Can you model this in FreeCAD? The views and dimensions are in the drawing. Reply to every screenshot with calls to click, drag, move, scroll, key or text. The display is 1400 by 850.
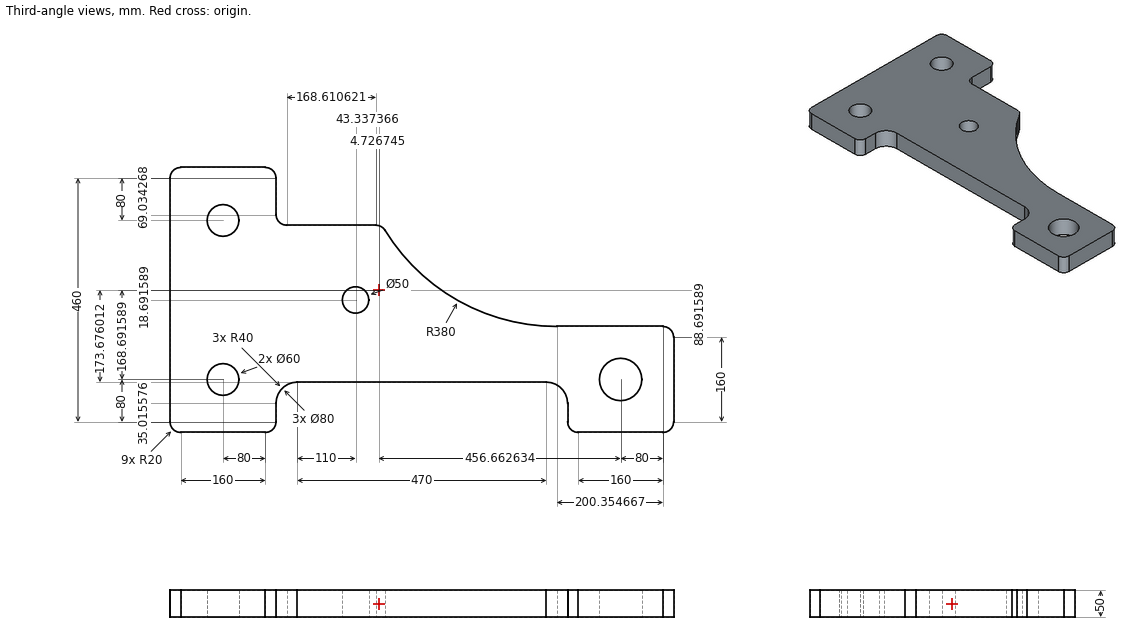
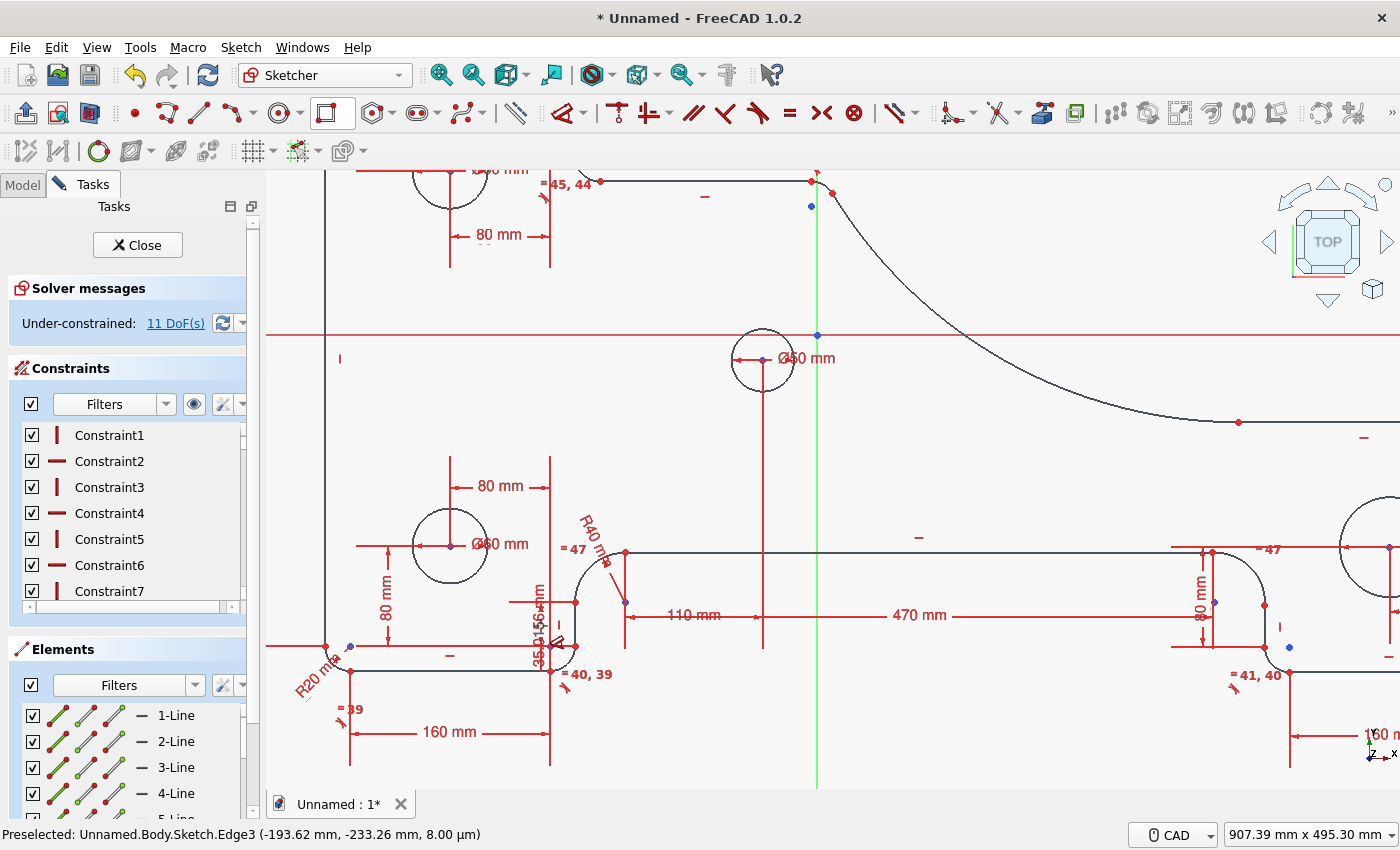
scroll(576, 626, down, 3)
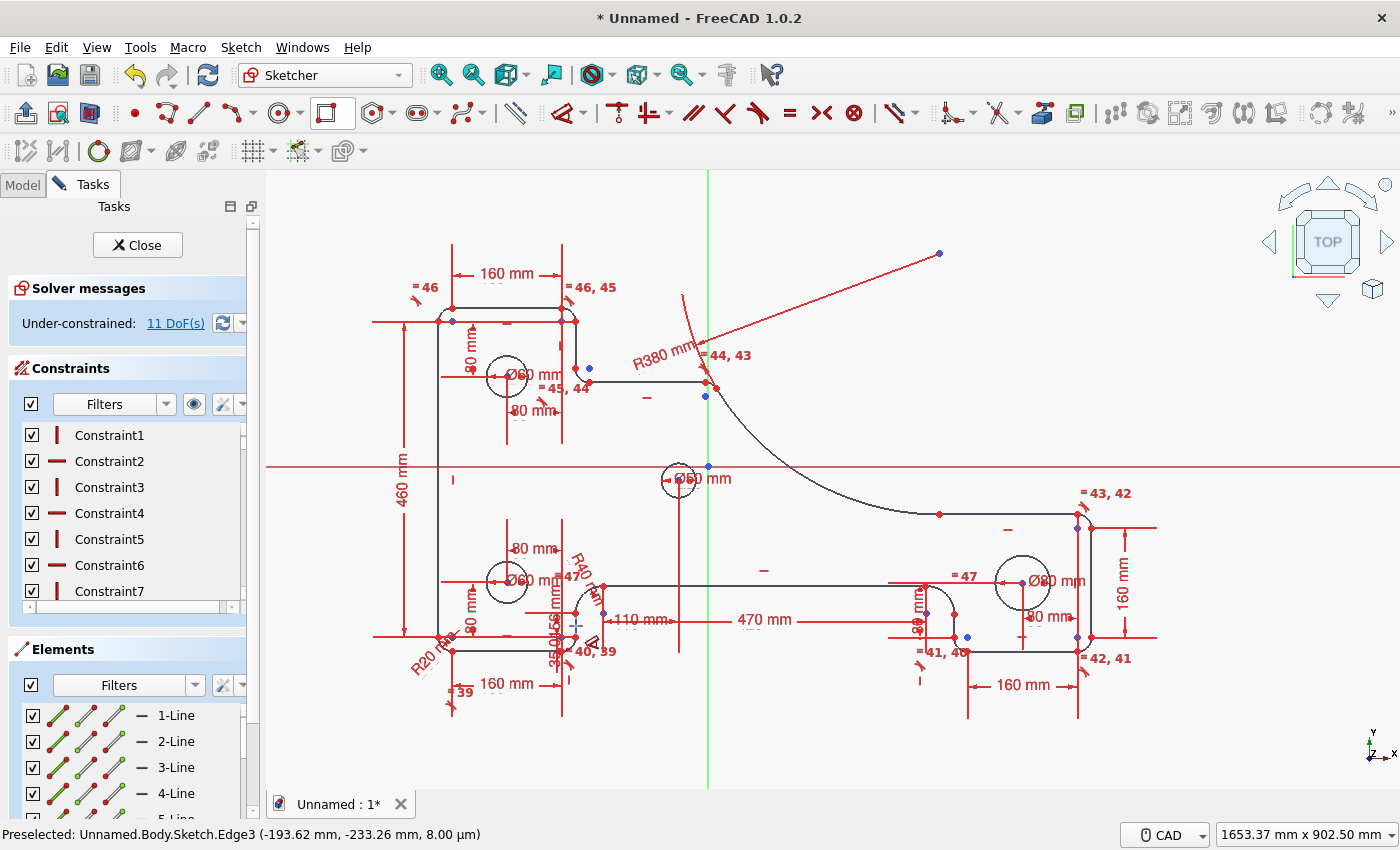
scroll(954, 622, up, 4)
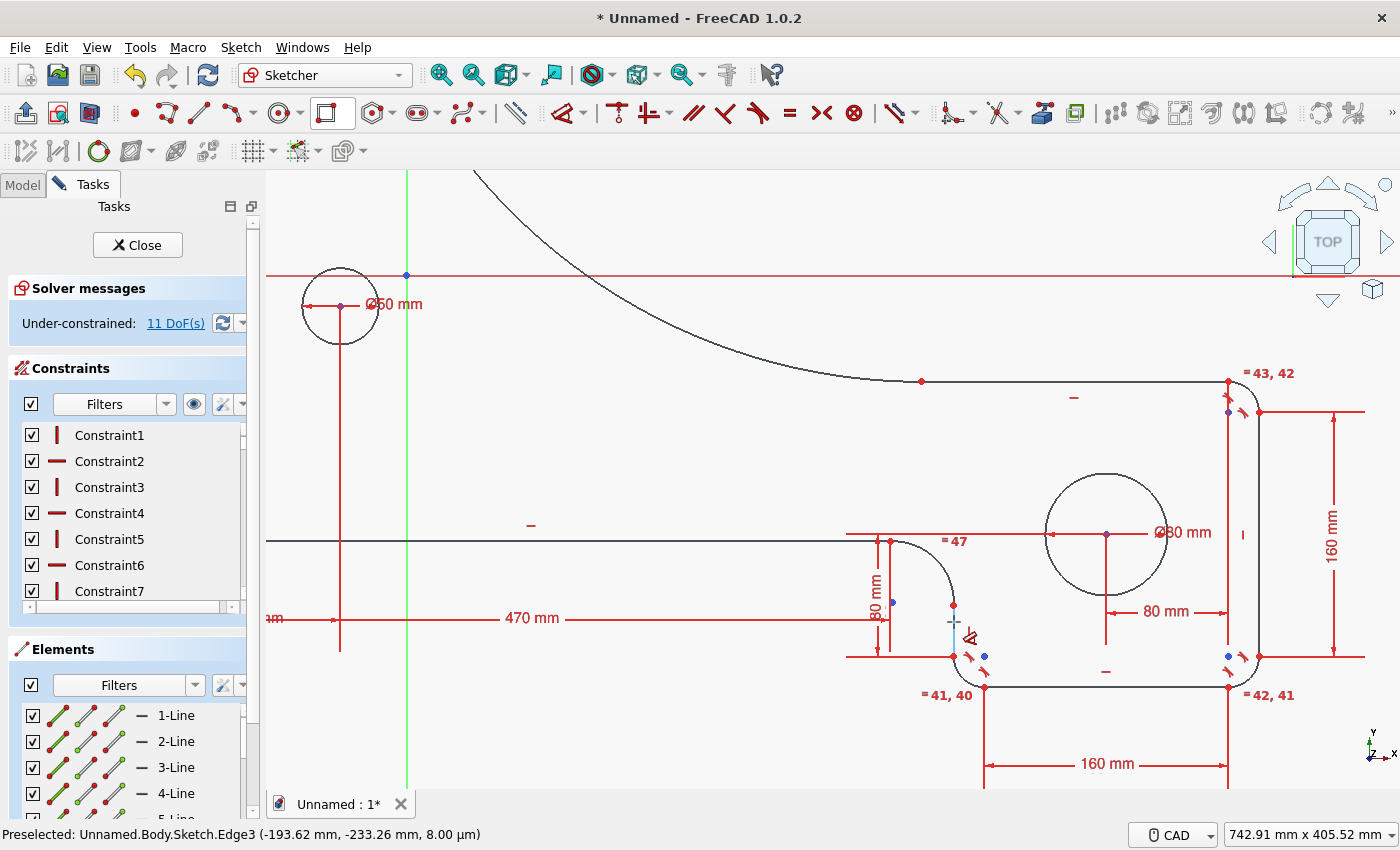
click(954, 621)
click(988, 631)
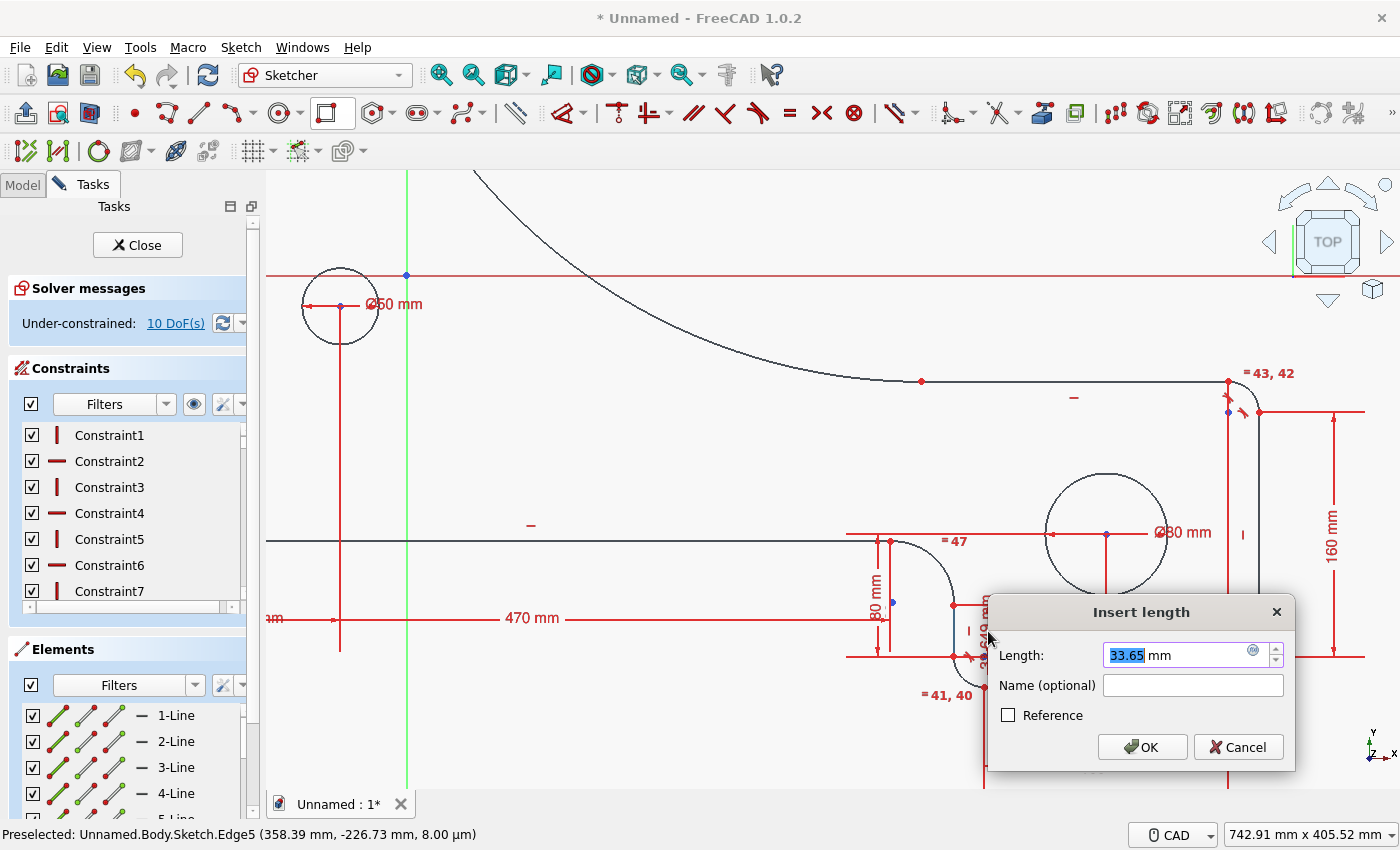
text(35.015576)
key(Return)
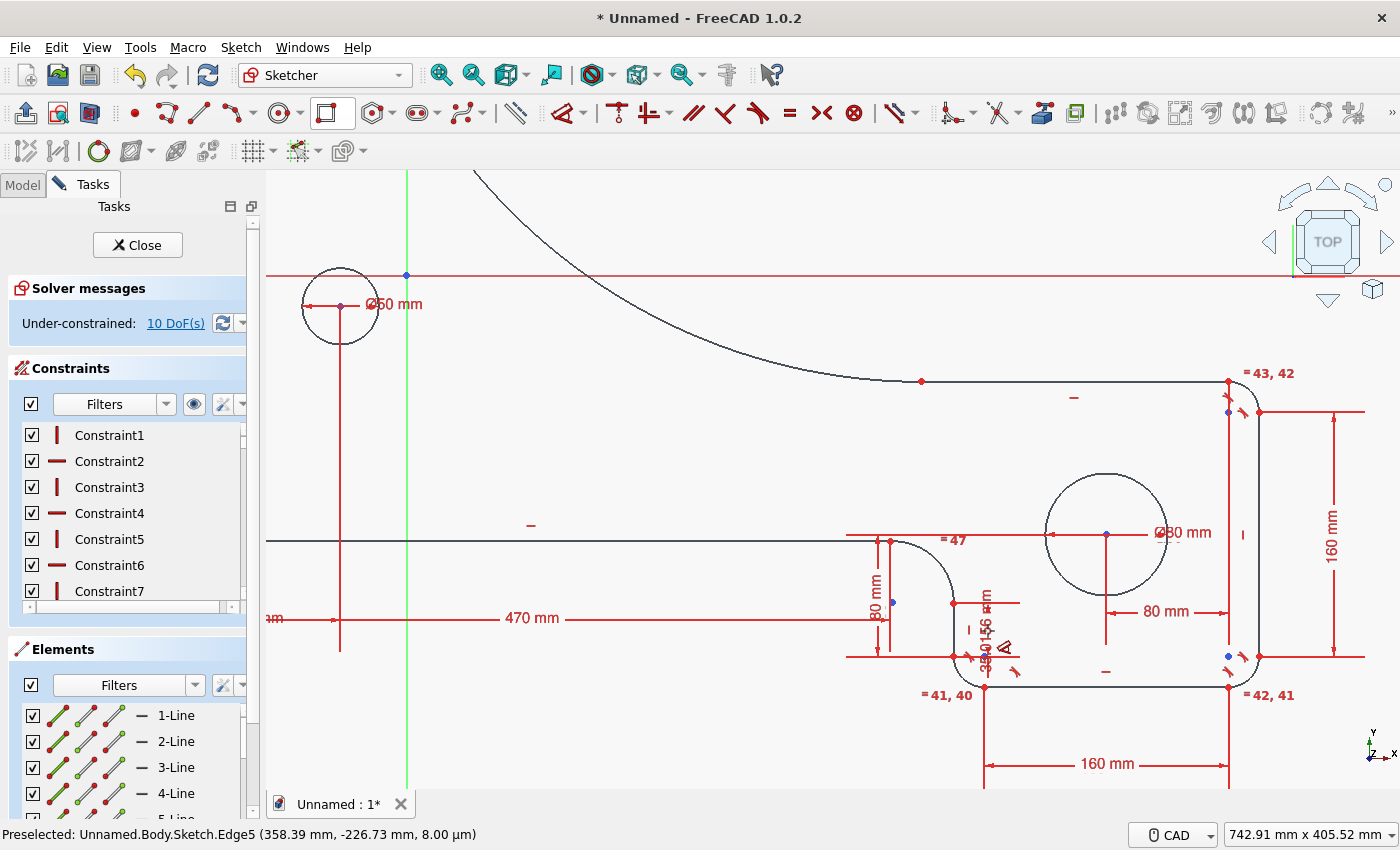
scroll(955, 622, down, 4)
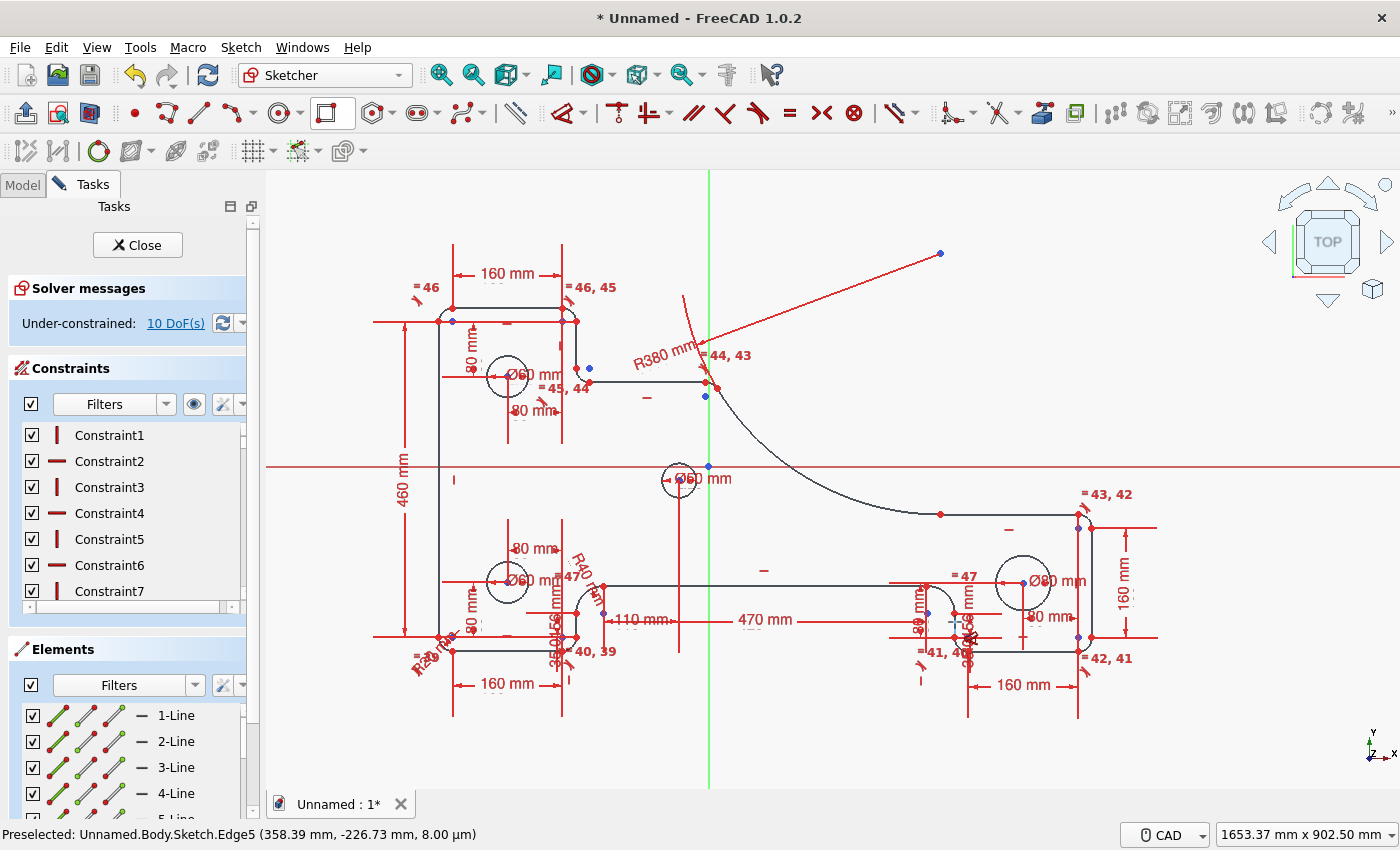
click(576, 355)
click(542, 329)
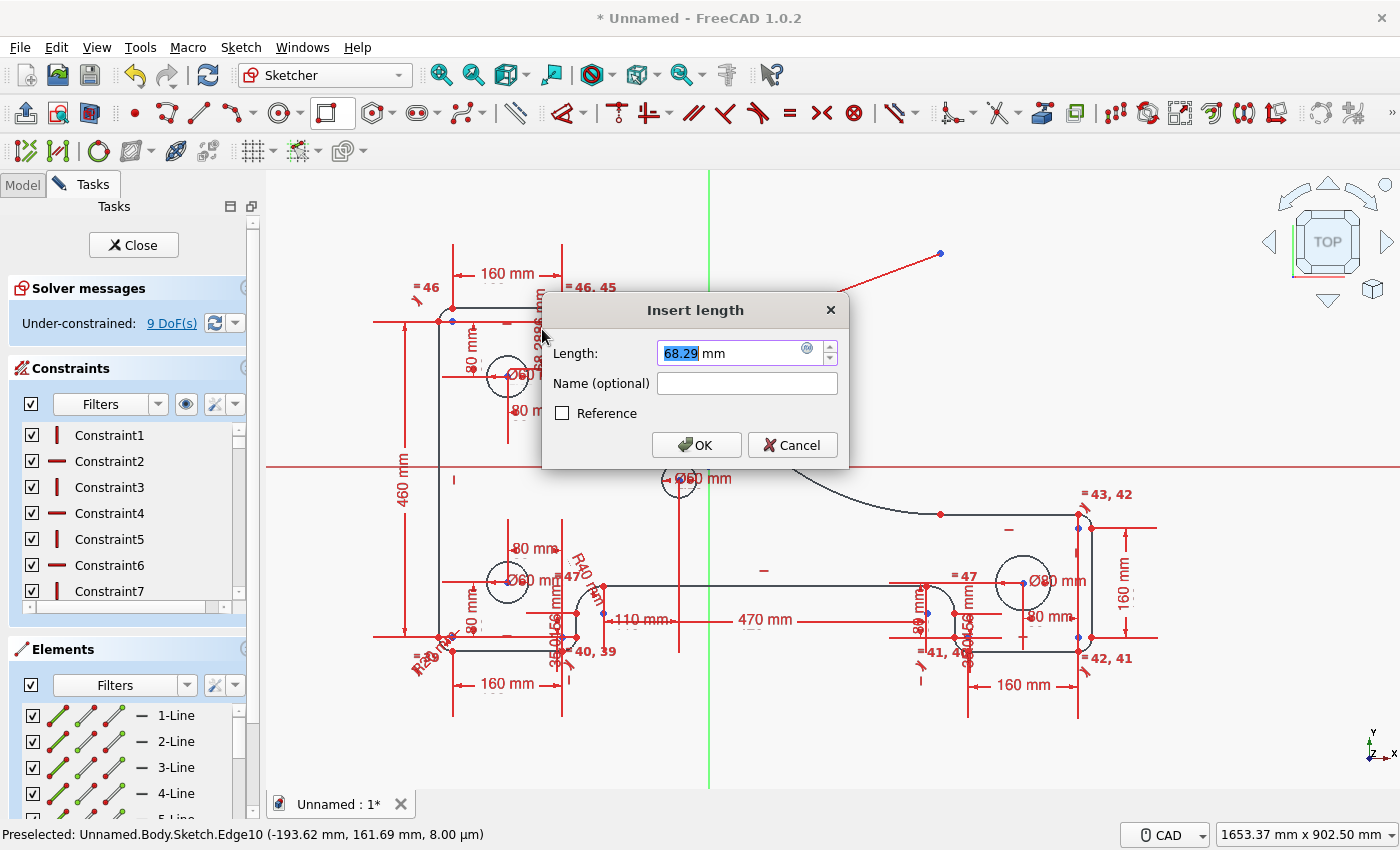
text(69.034268)
key(Return)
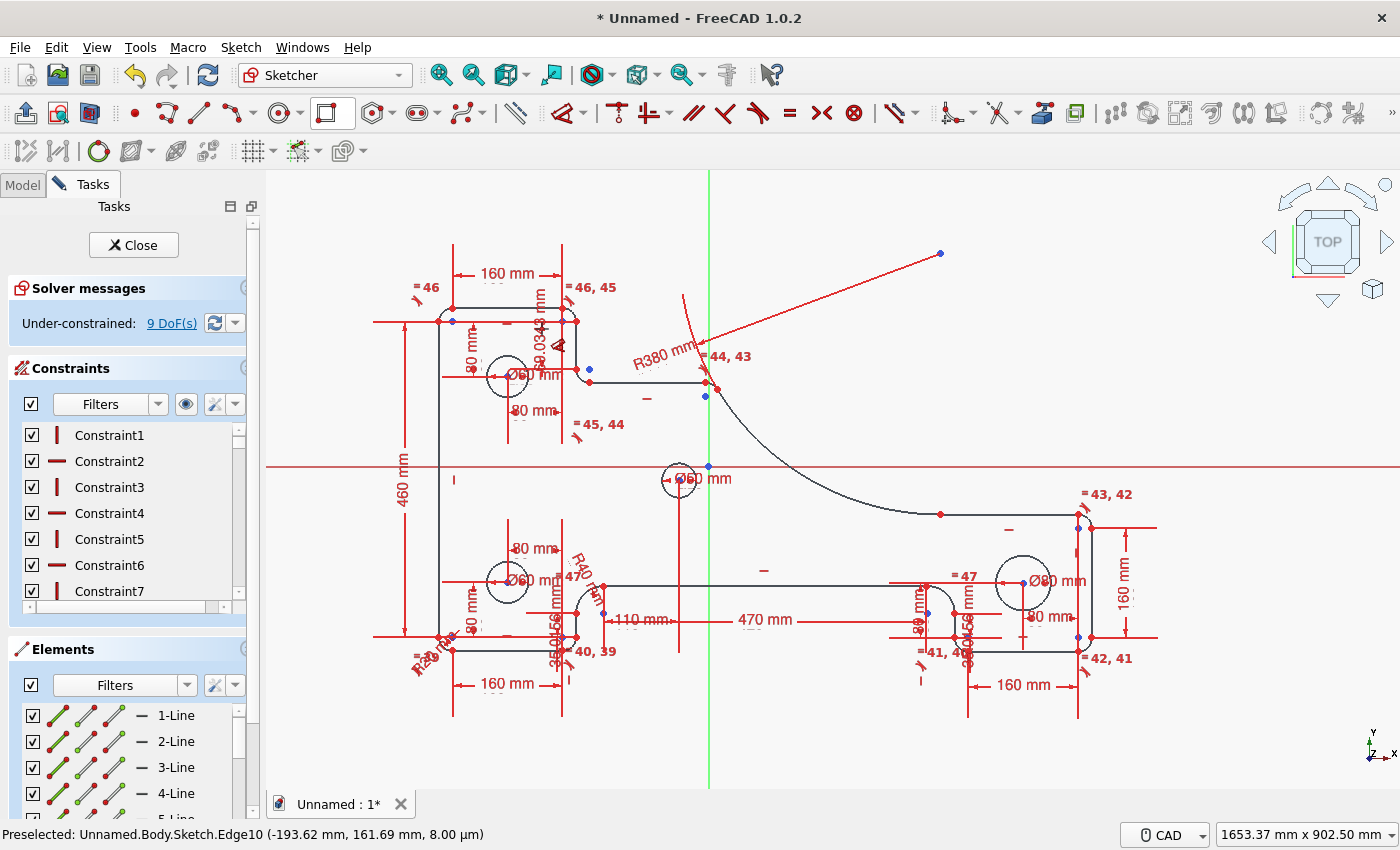
scroll(706, 383, up, 13)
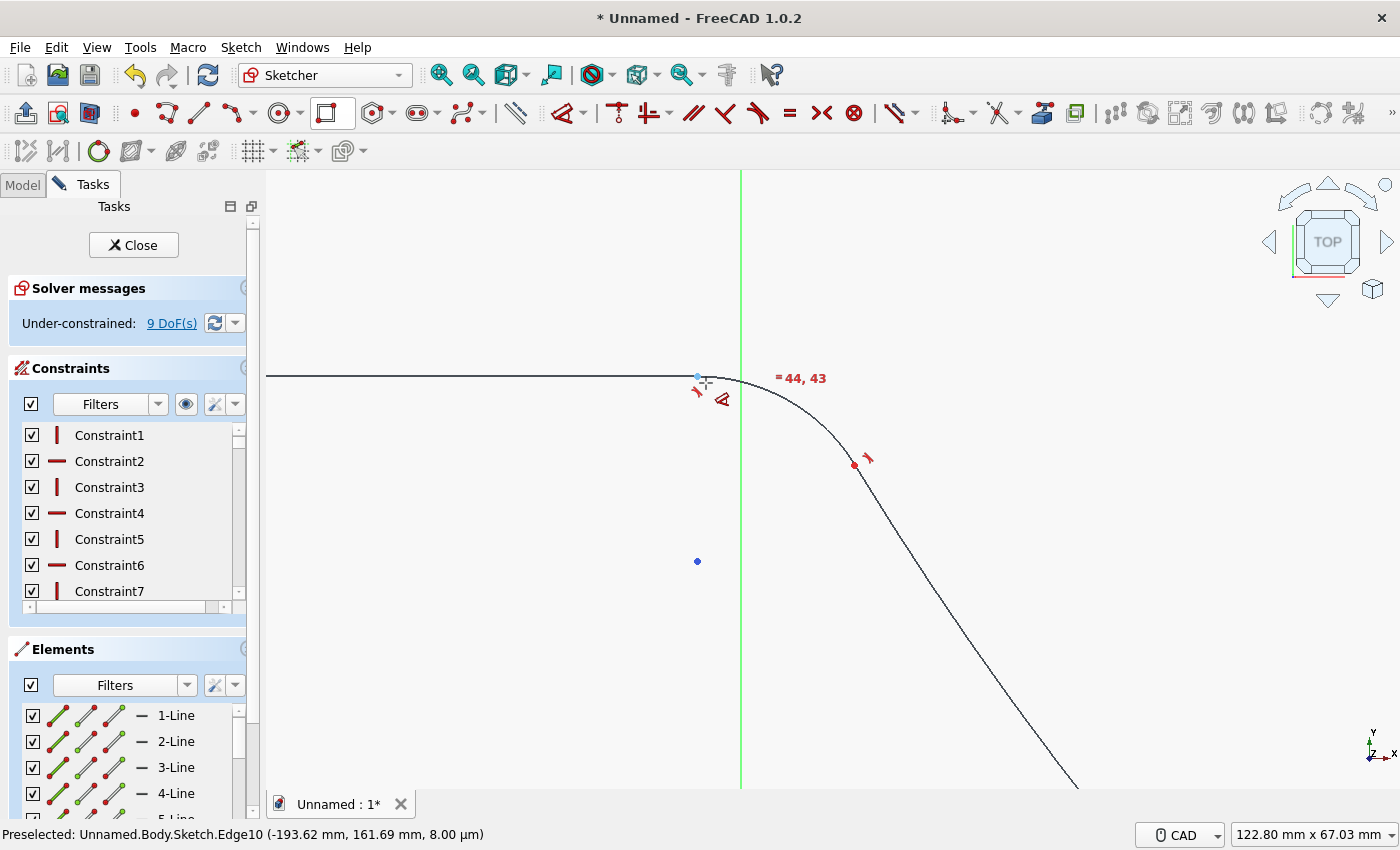
click(697, 376)
click(719, 342)